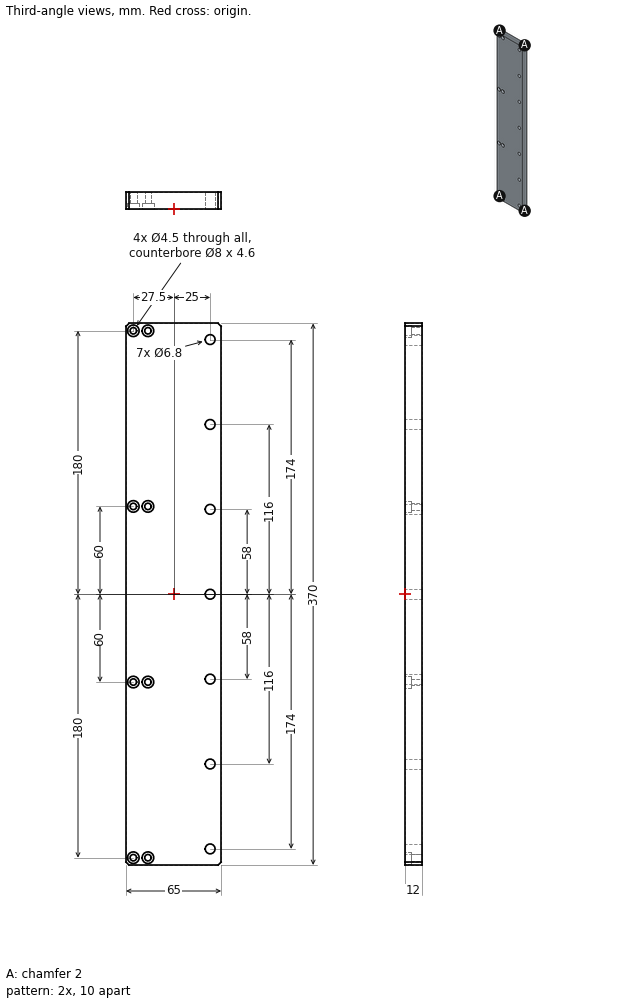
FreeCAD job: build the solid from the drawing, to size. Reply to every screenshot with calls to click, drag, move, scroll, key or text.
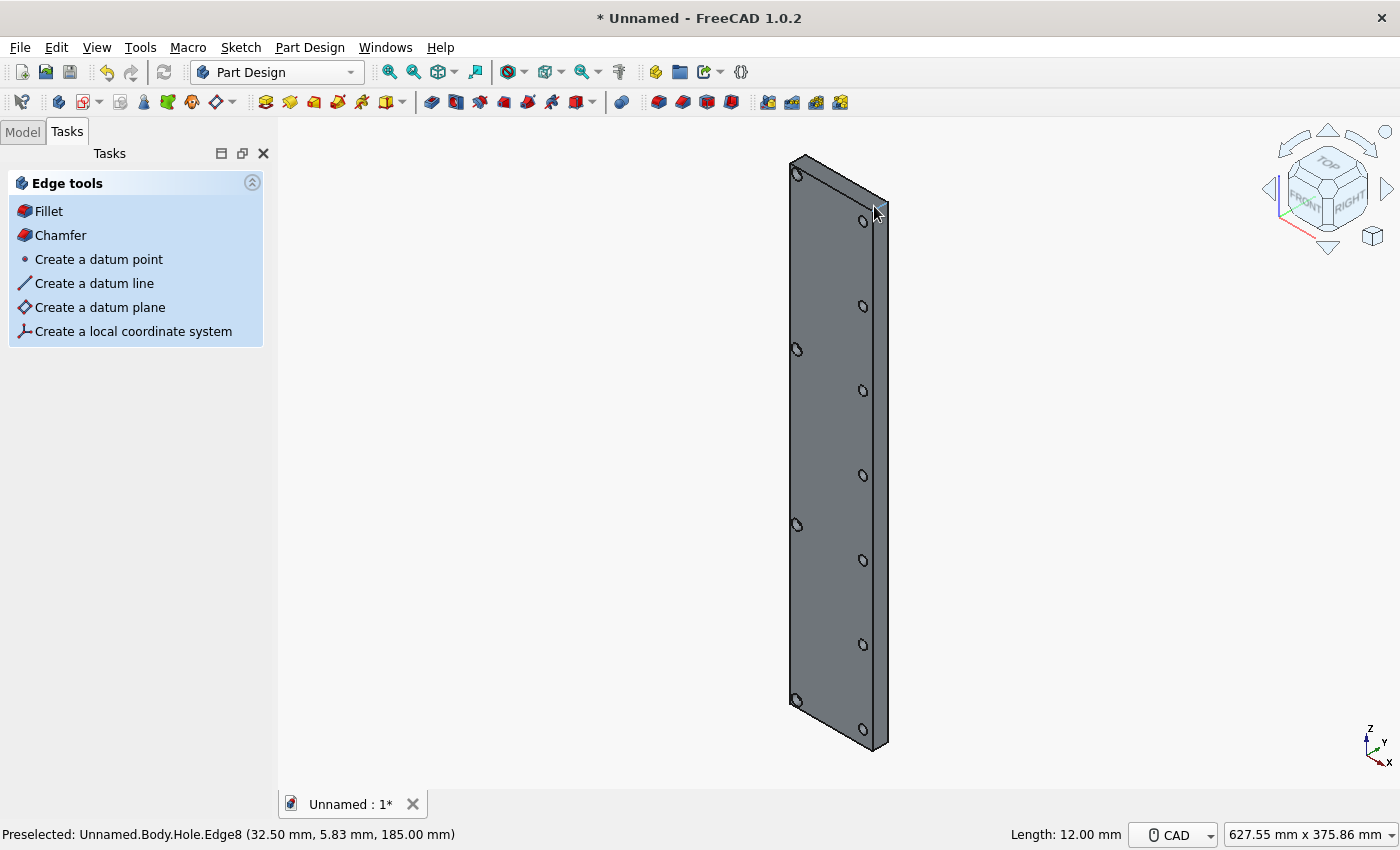
scroll(798, 158, up, 4)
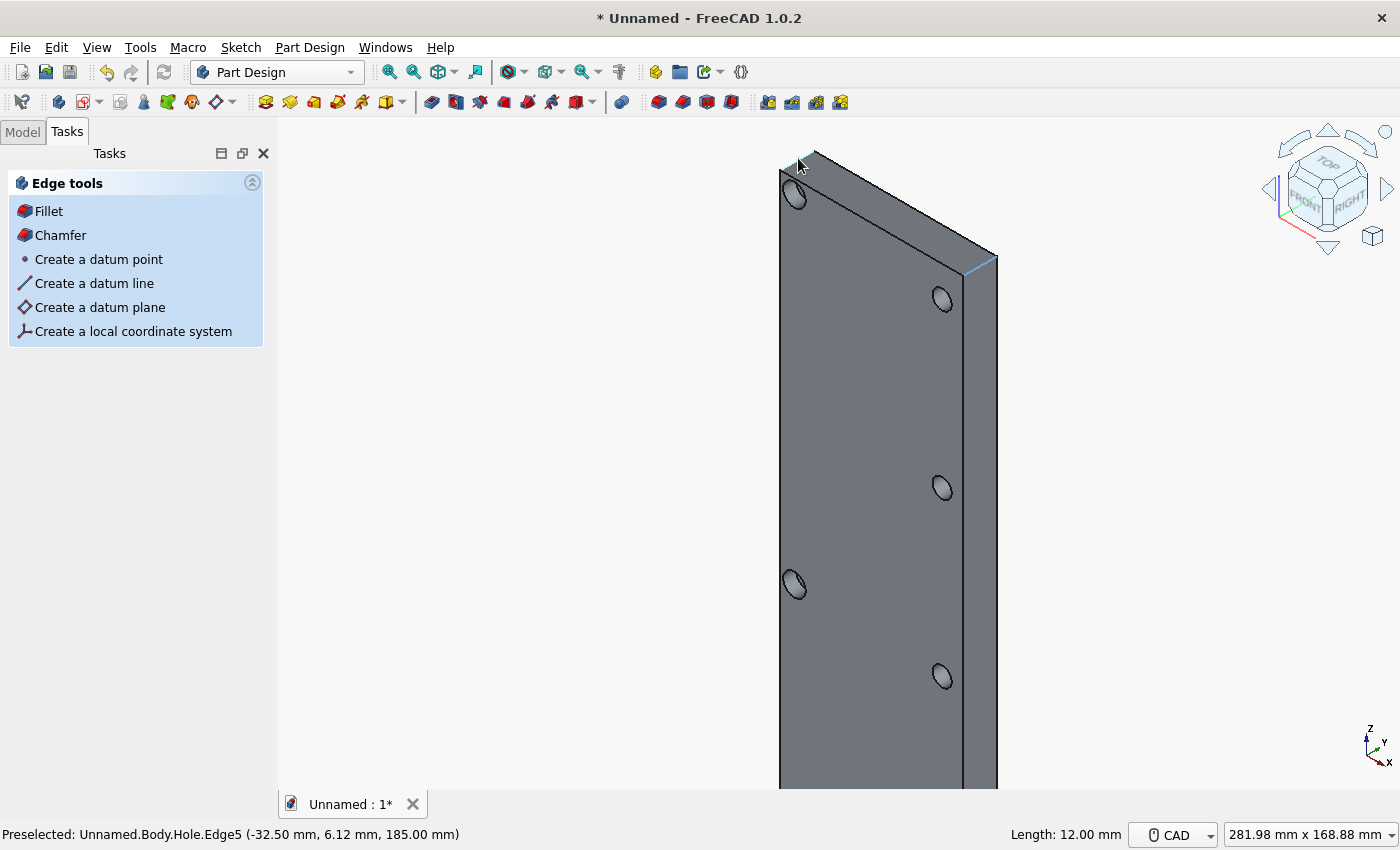
key(v)
key(f)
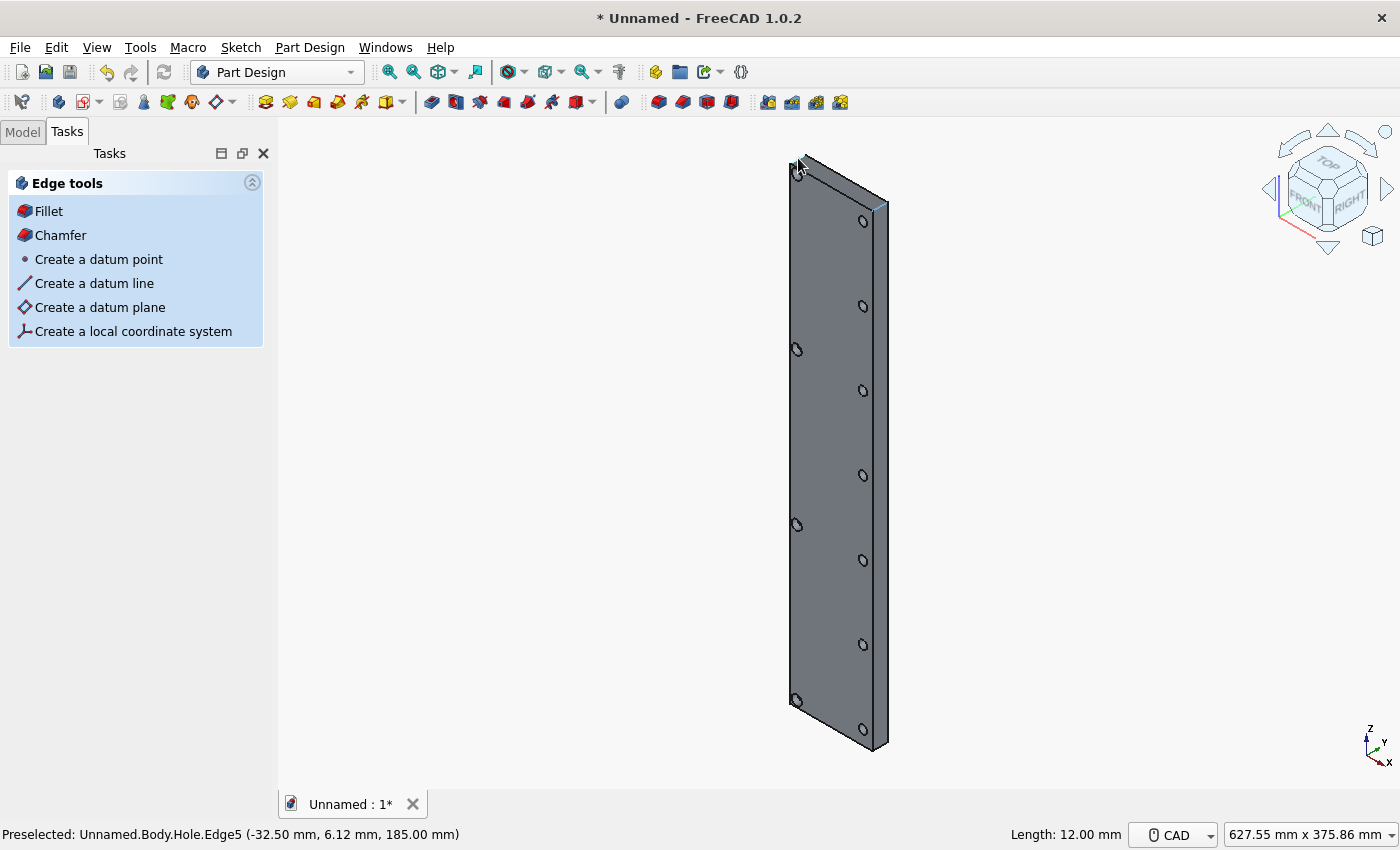
key(2)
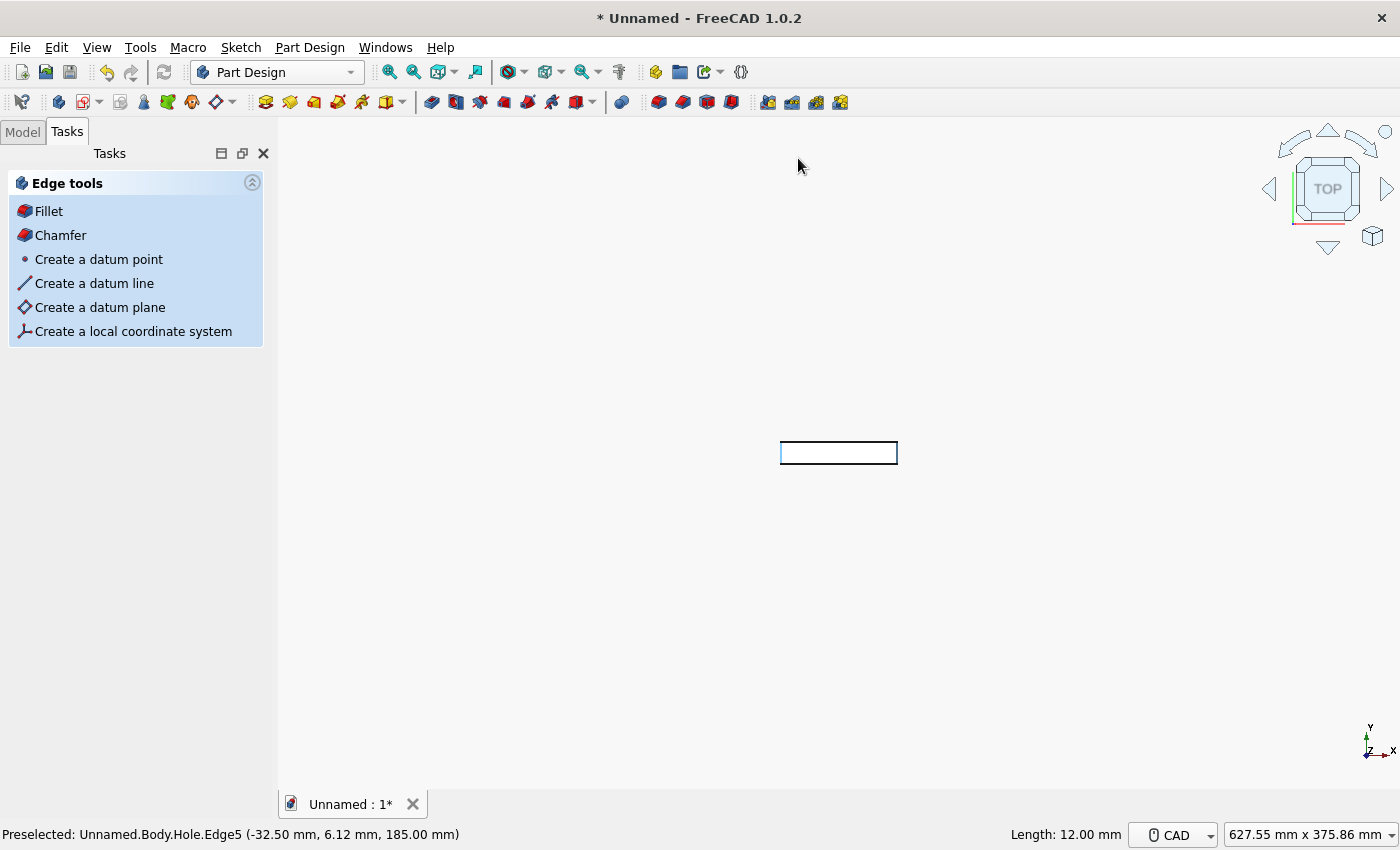
click(390, 72)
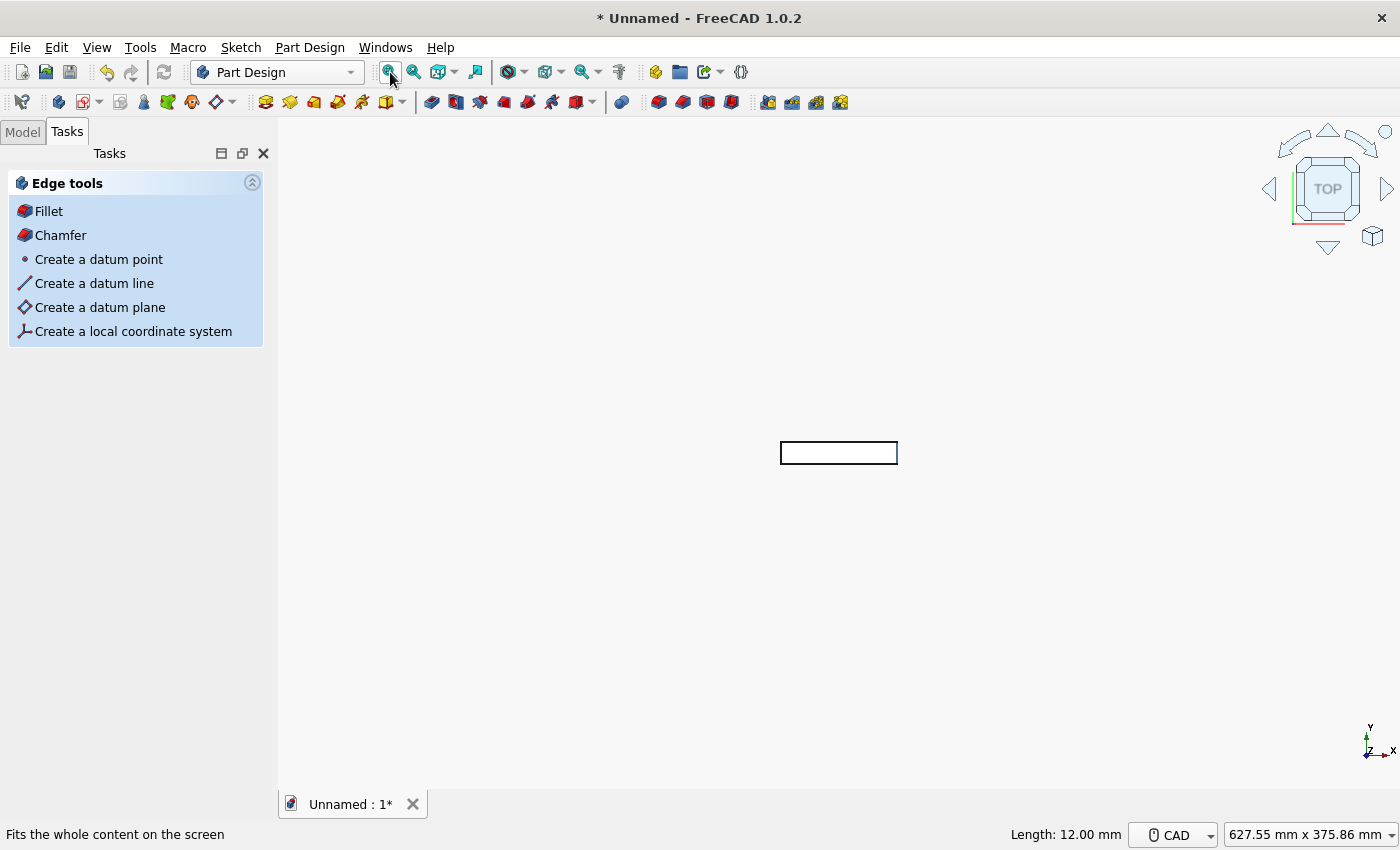
click(781, 452, ctrl)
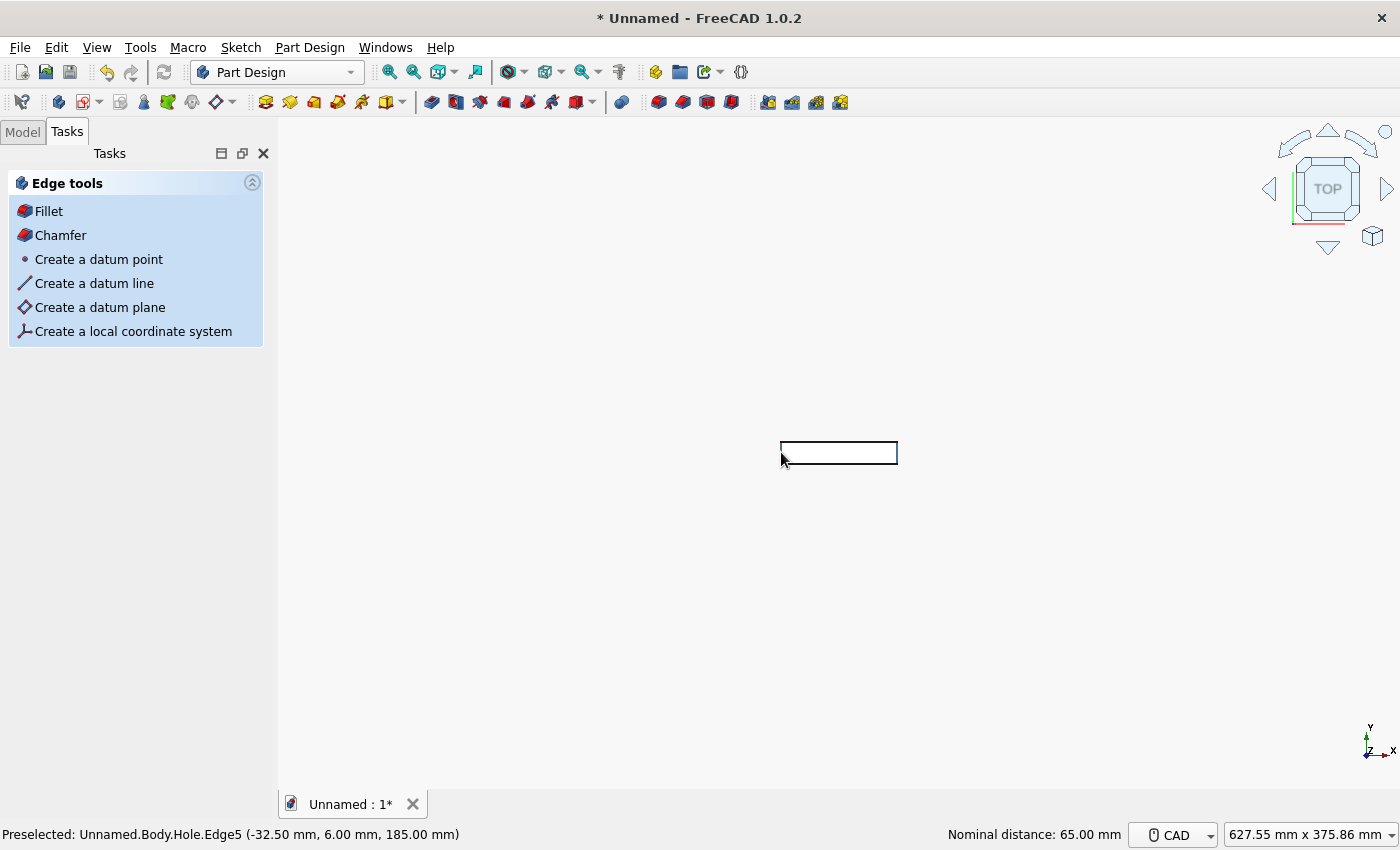
scroll(781, 452, up, 4)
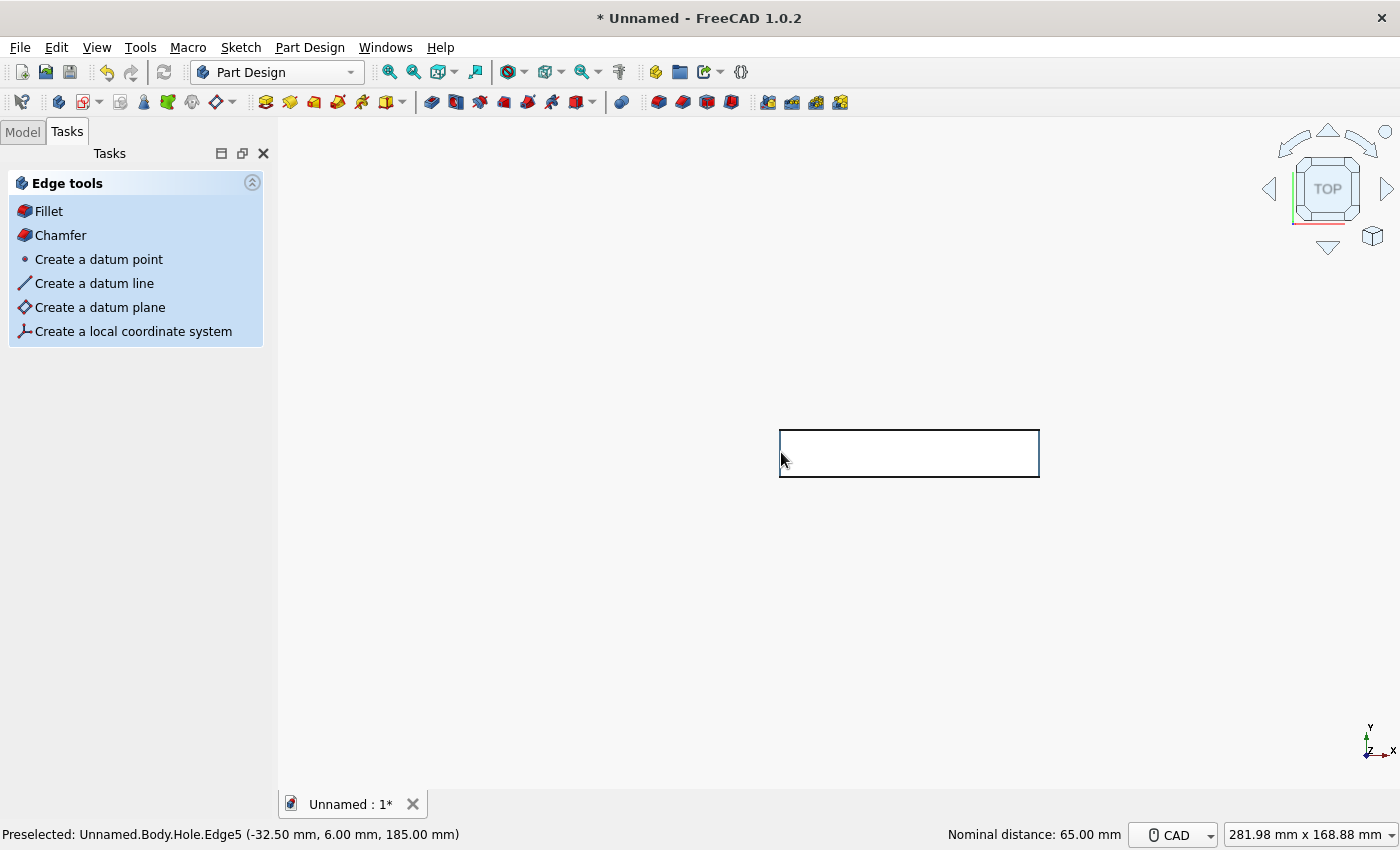
click(390, 72)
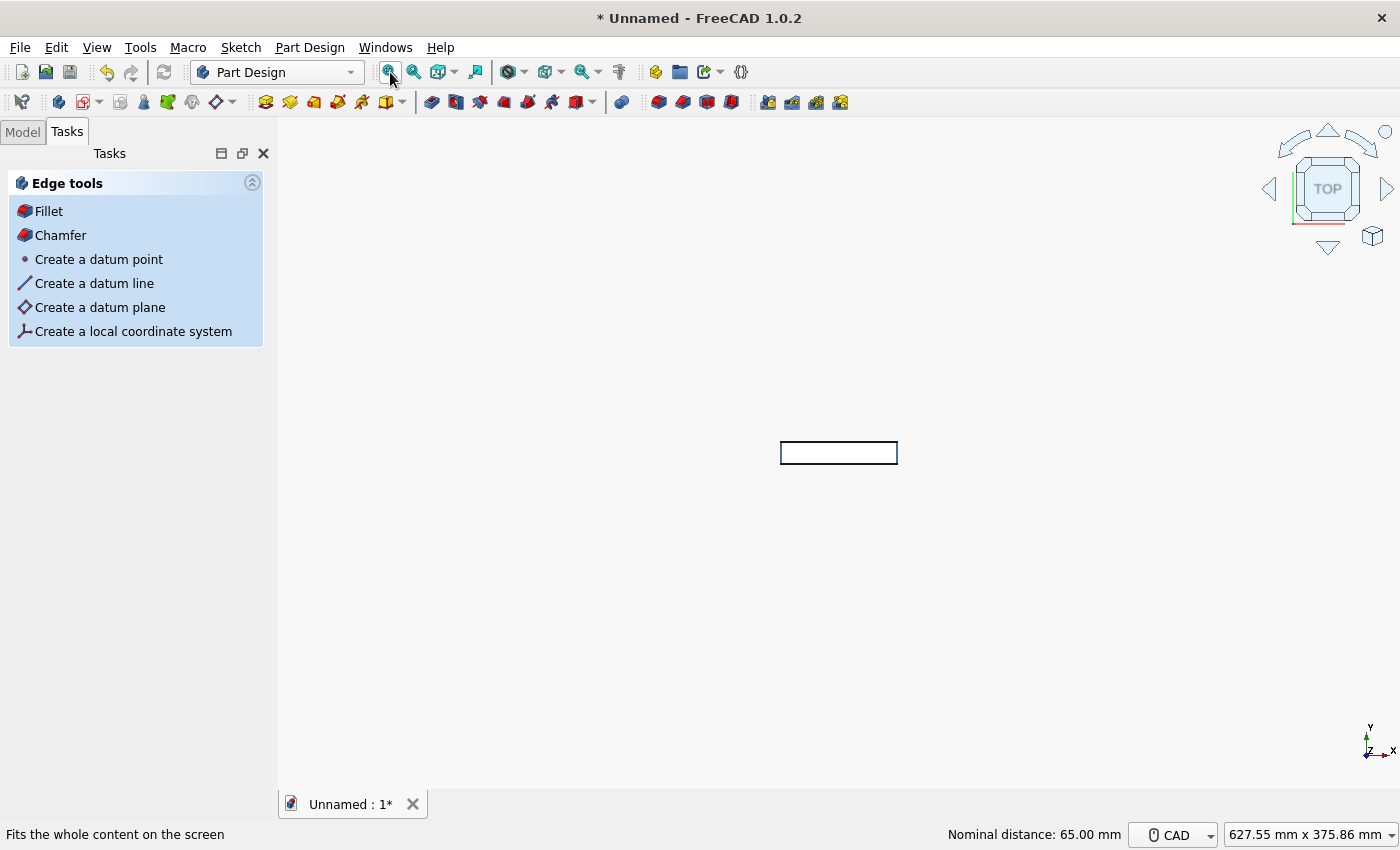
key(0)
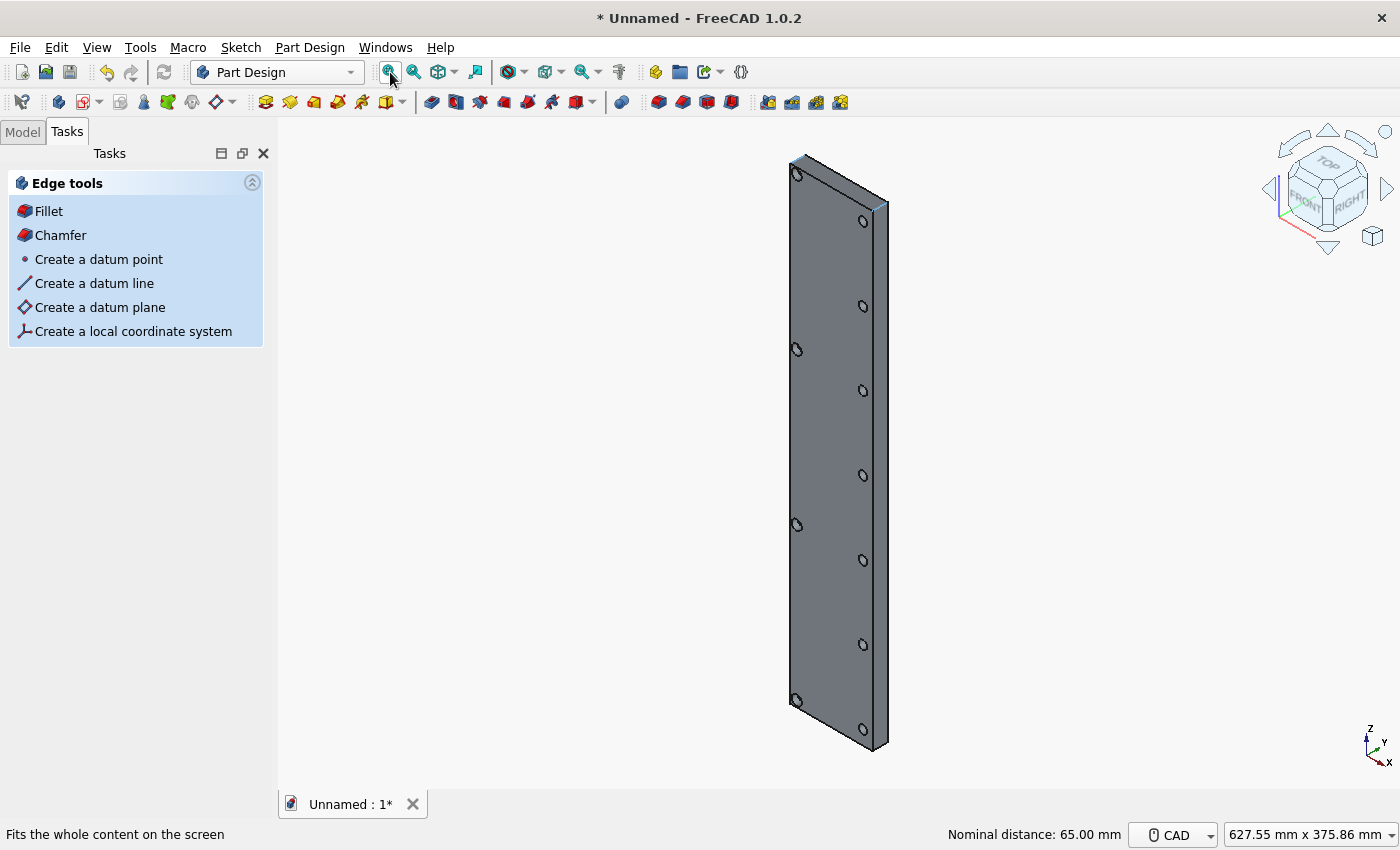
scroll(798, 698, up, 4)